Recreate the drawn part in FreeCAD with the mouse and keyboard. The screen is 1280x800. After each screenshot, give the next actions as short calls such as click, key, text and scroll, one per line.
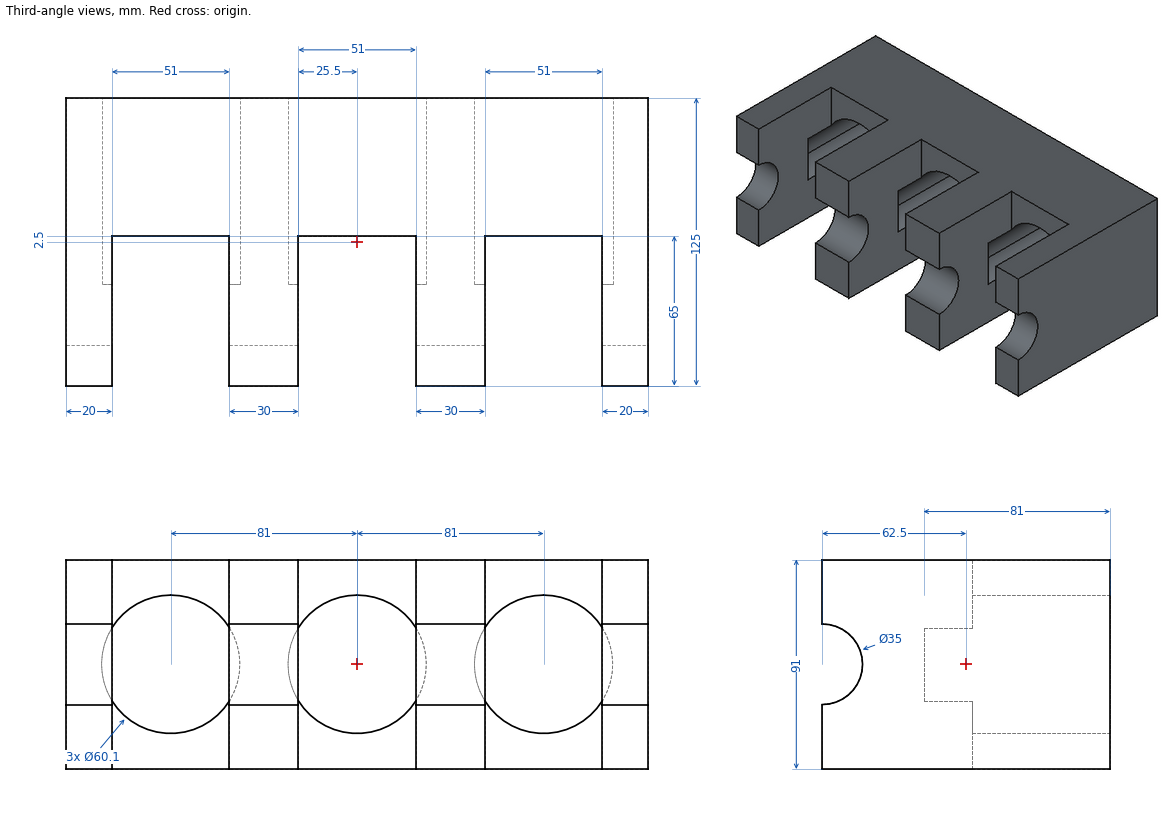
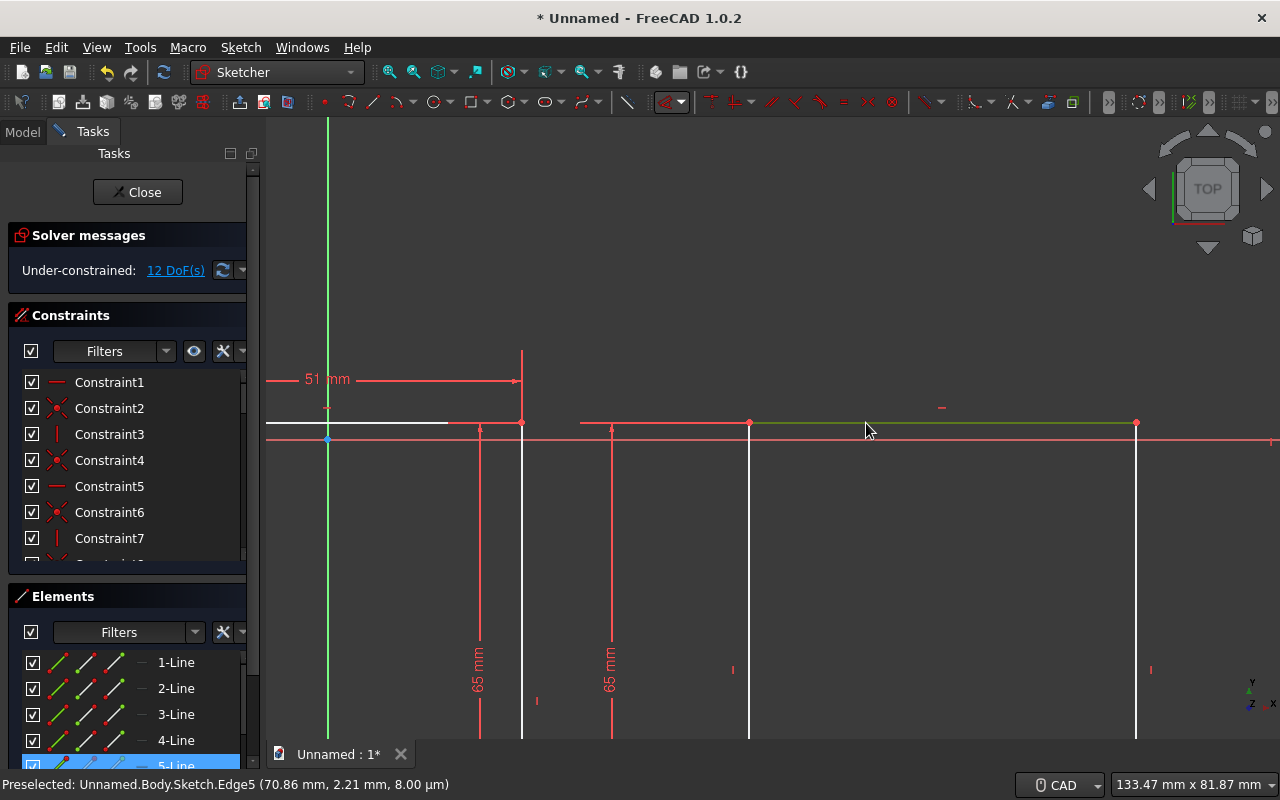
key(l)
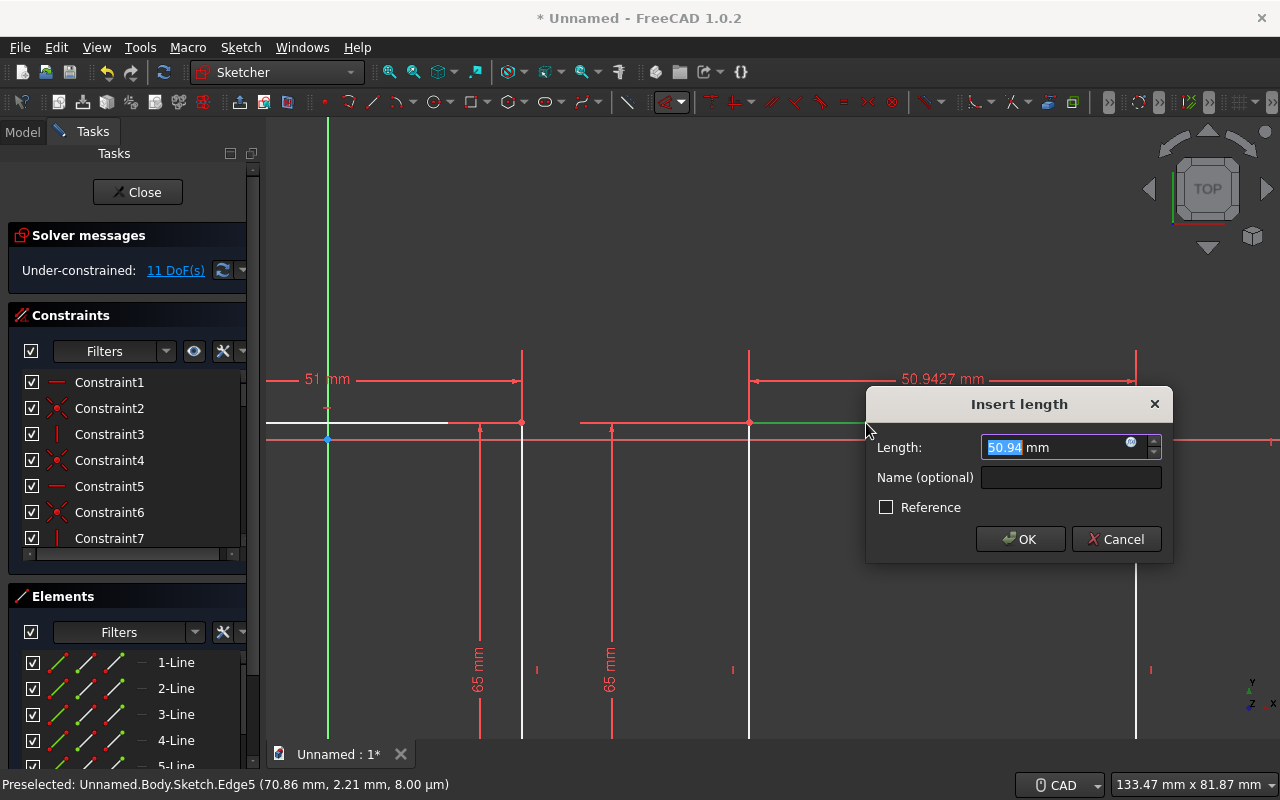
text(51)
key(Return)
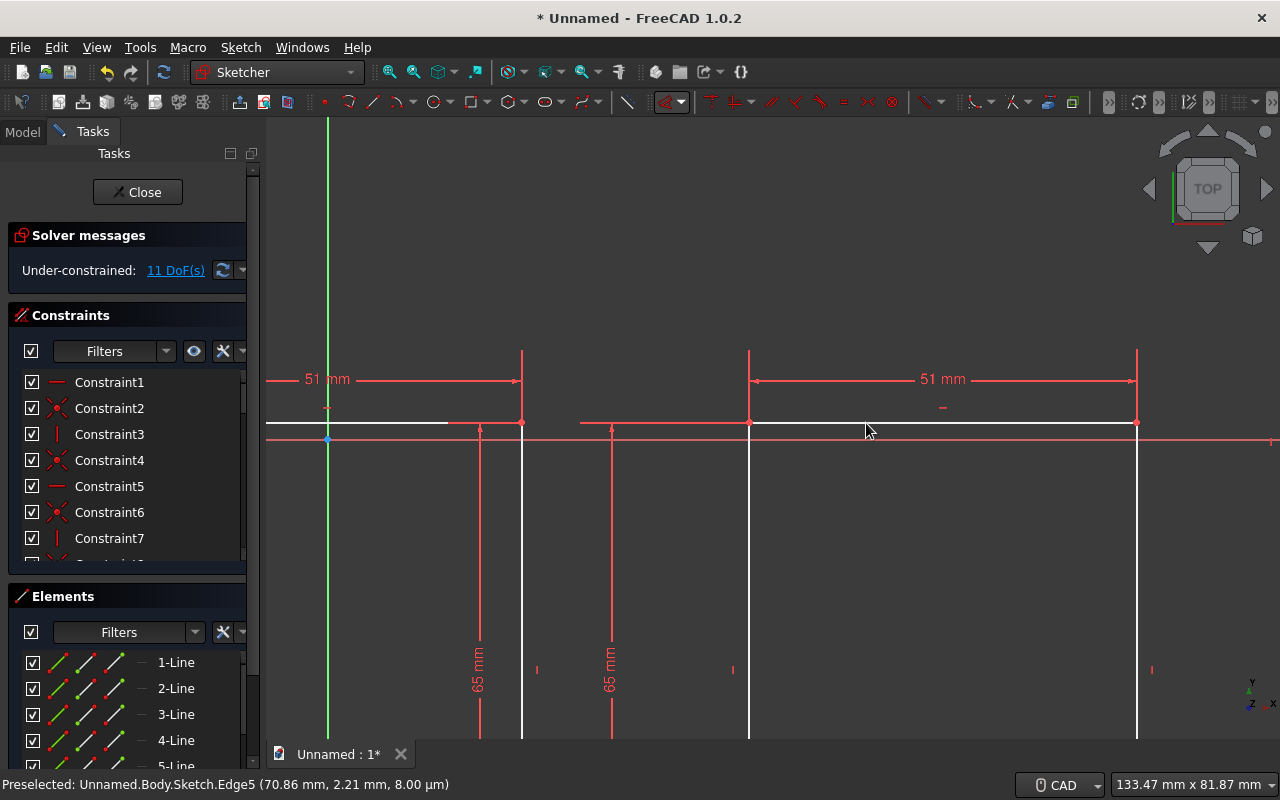
scroll(867, 423, down, 6)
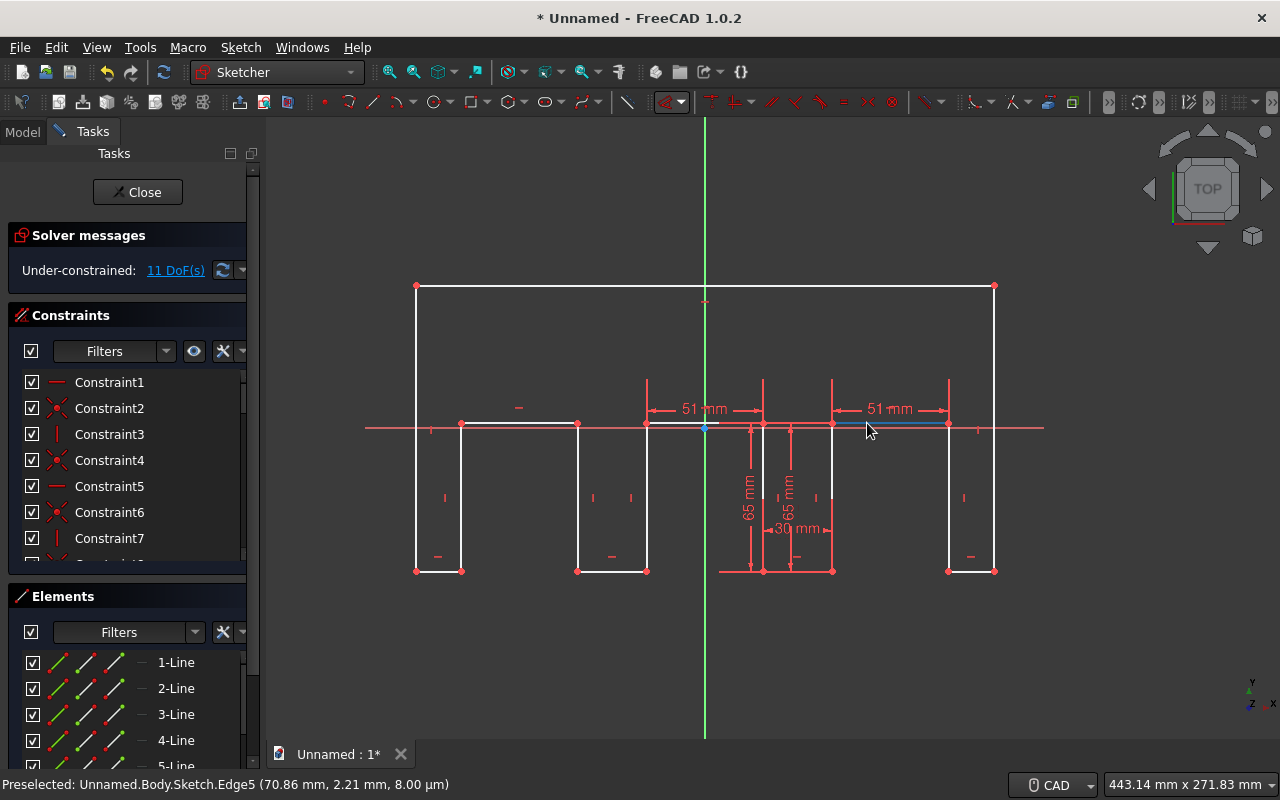
click(949, 468)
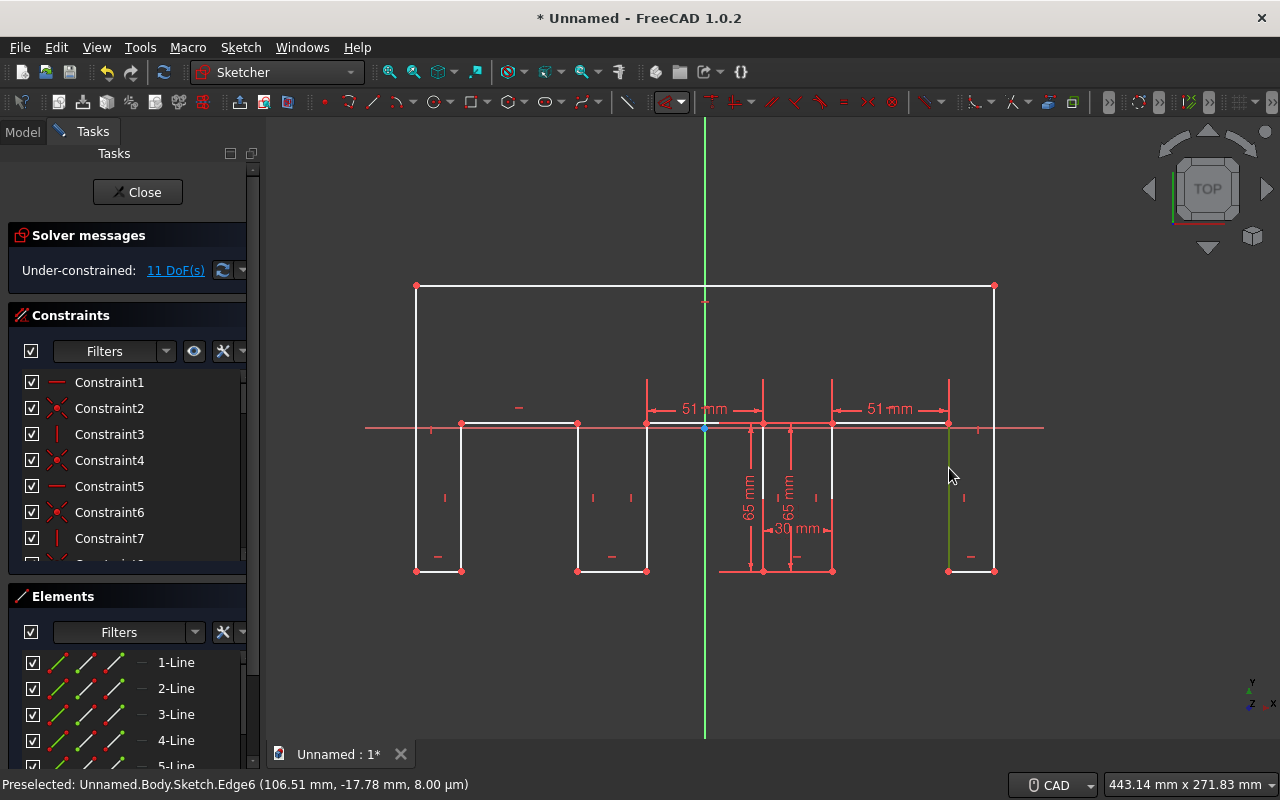
click(684, 102)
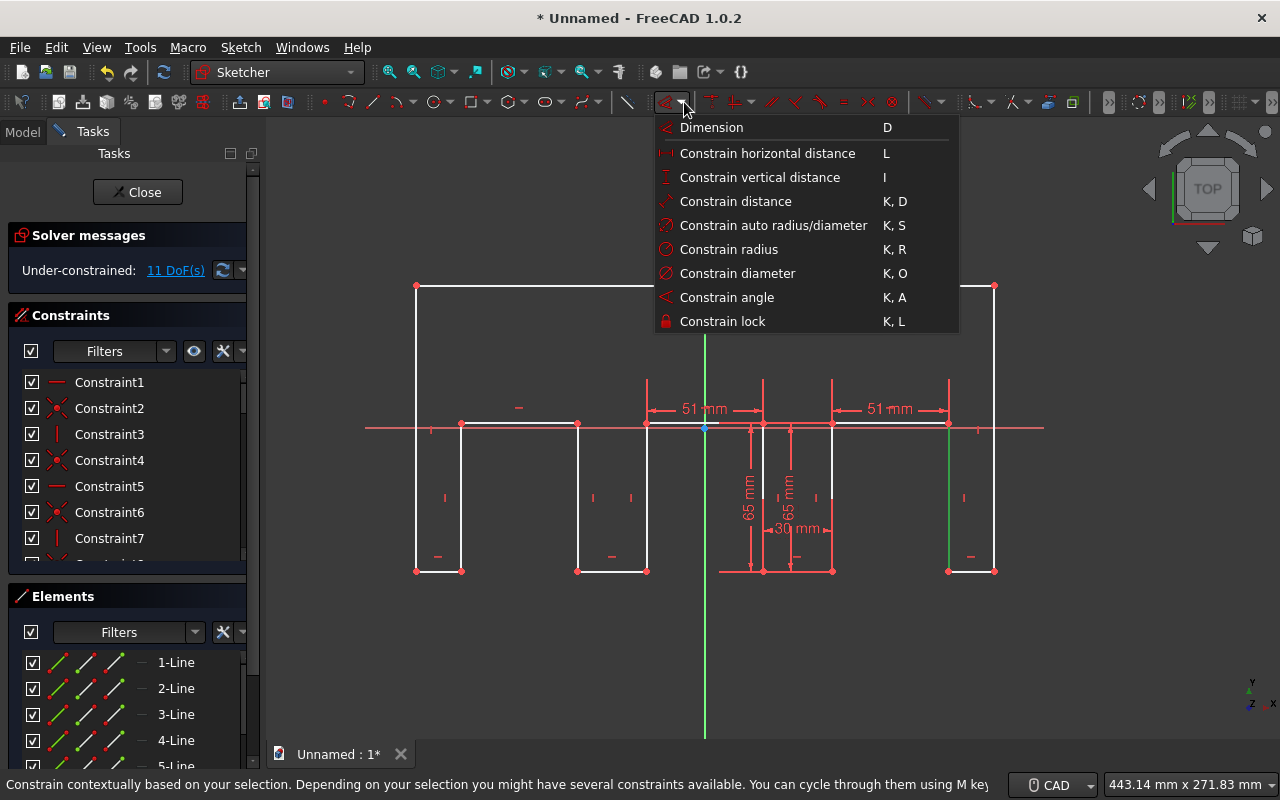
click(807, 177)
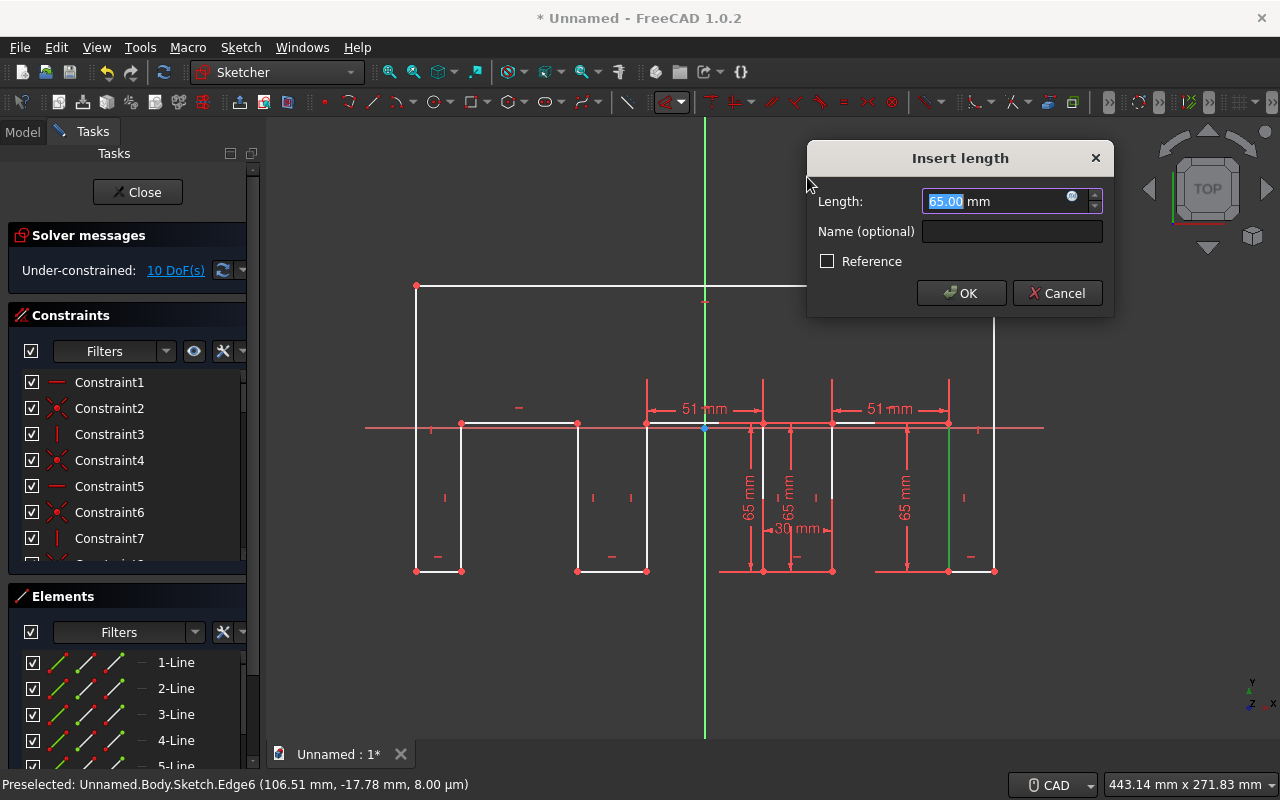
text(65)
key(Return)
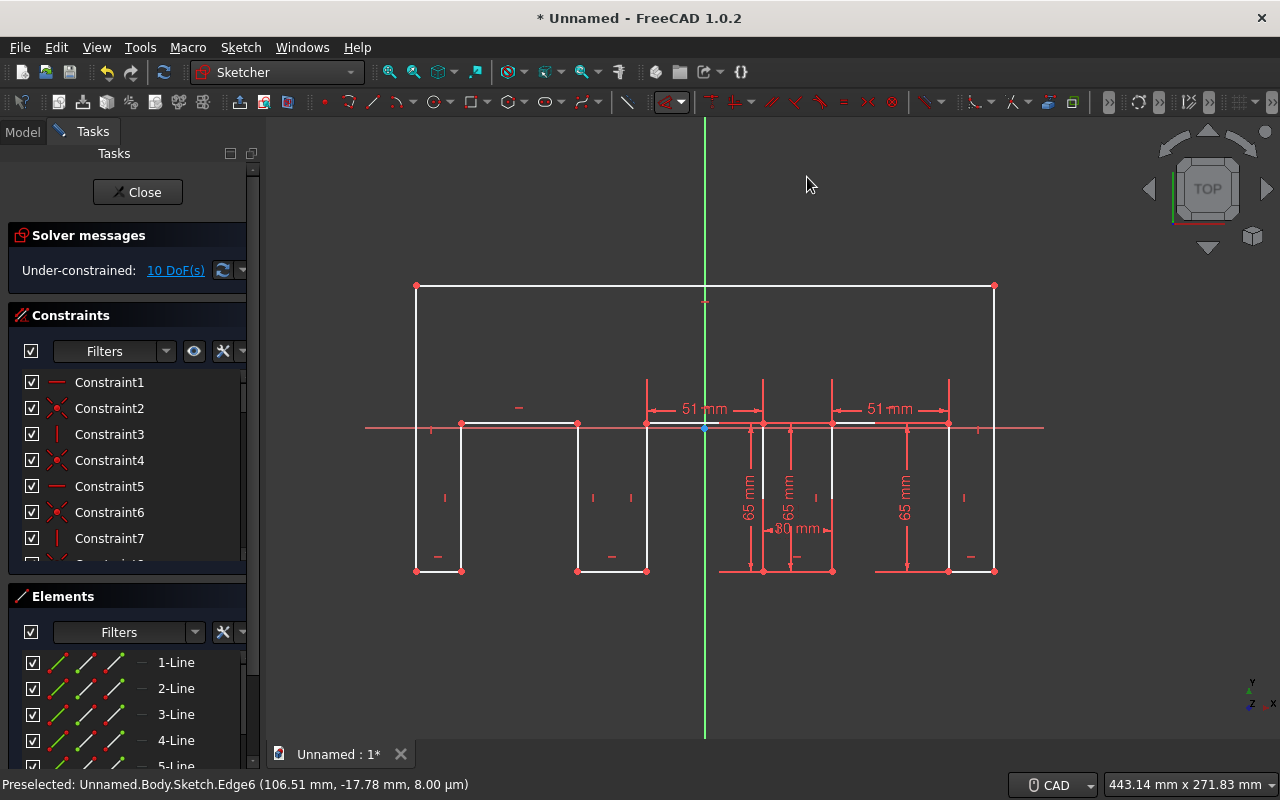
click(962, 572)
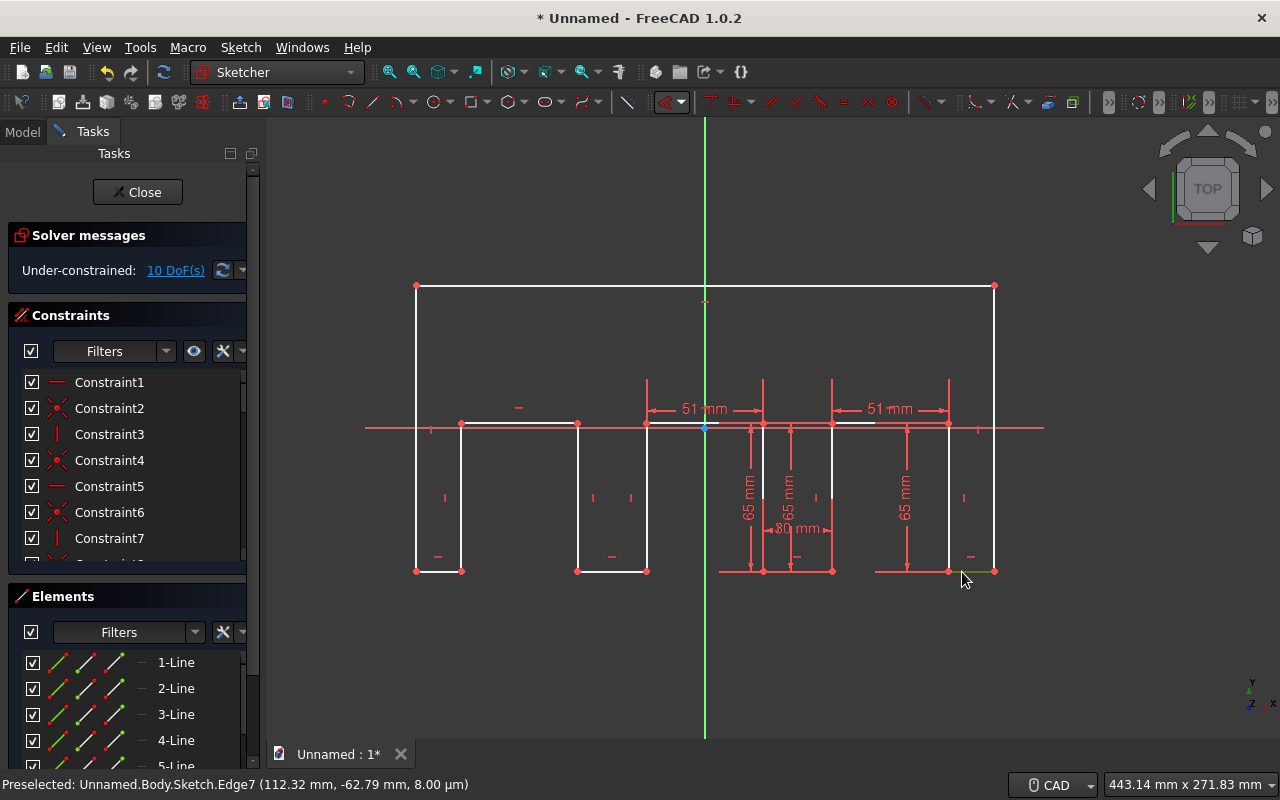
click(684, 102)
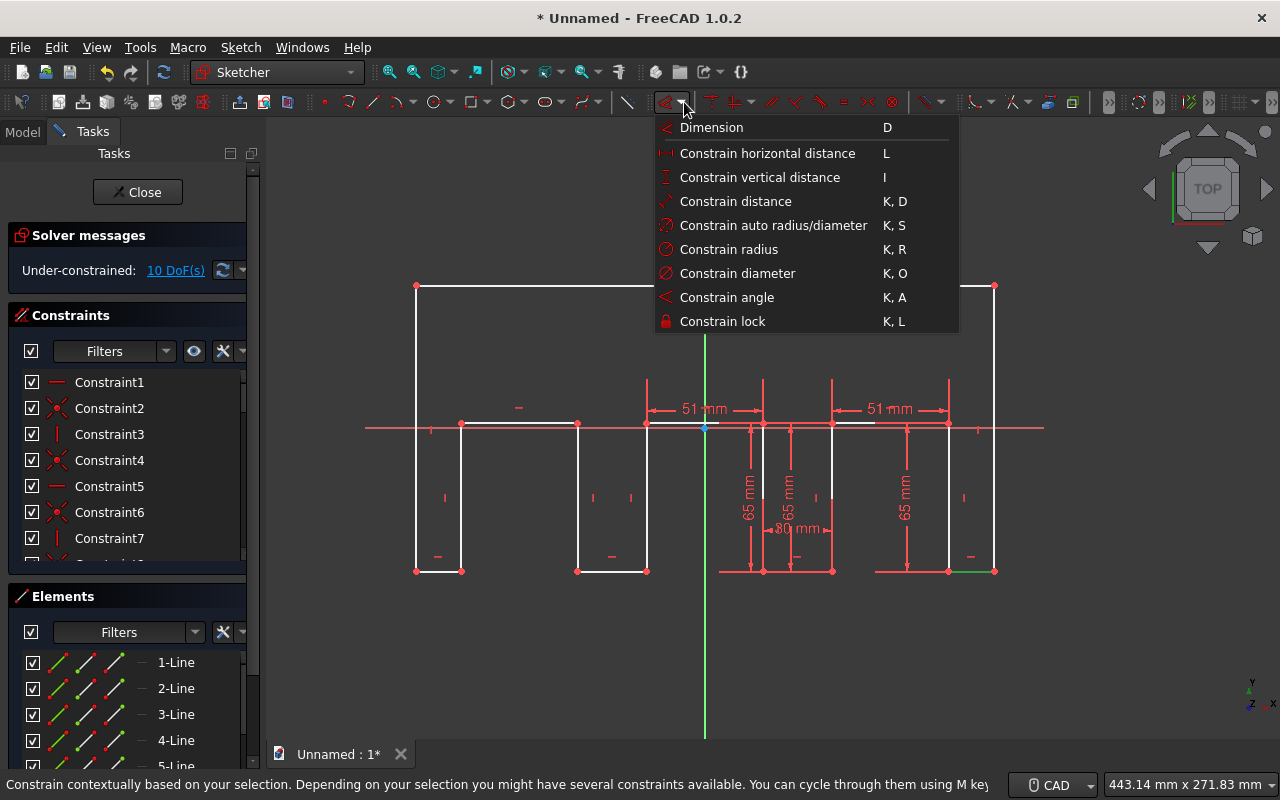
click(807, 153)